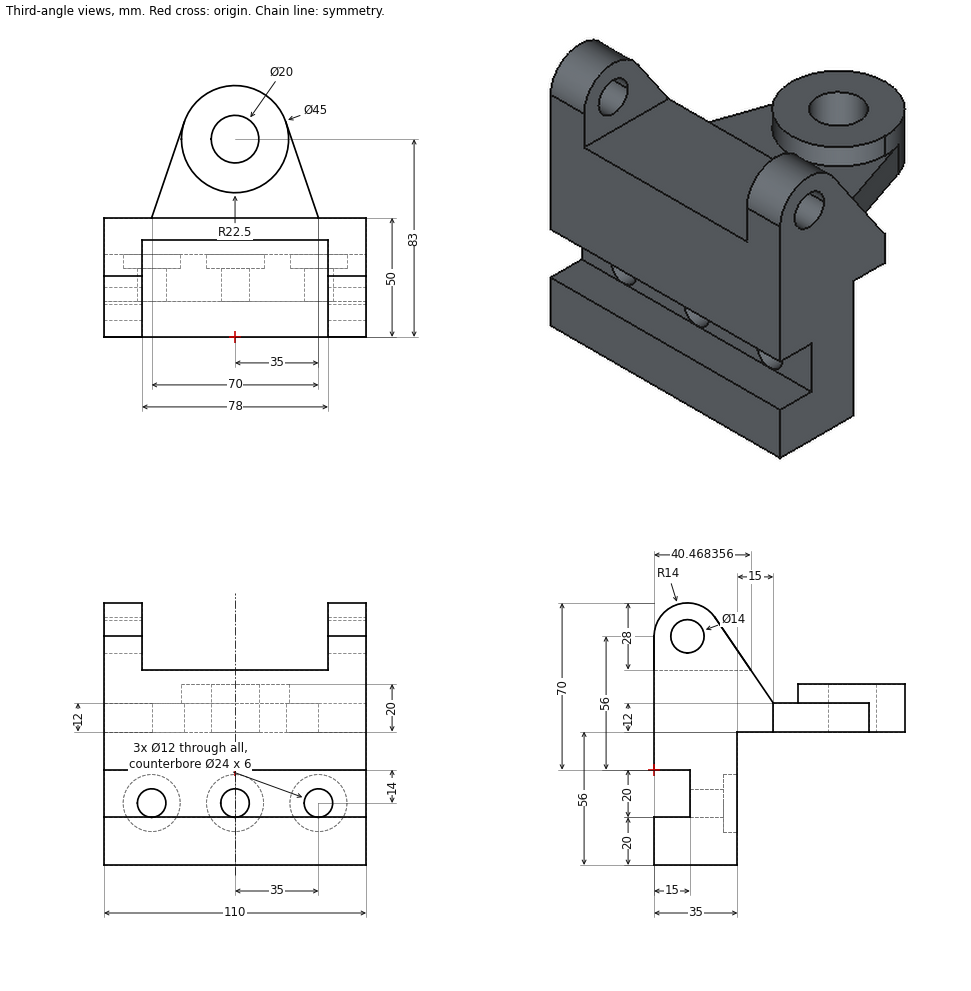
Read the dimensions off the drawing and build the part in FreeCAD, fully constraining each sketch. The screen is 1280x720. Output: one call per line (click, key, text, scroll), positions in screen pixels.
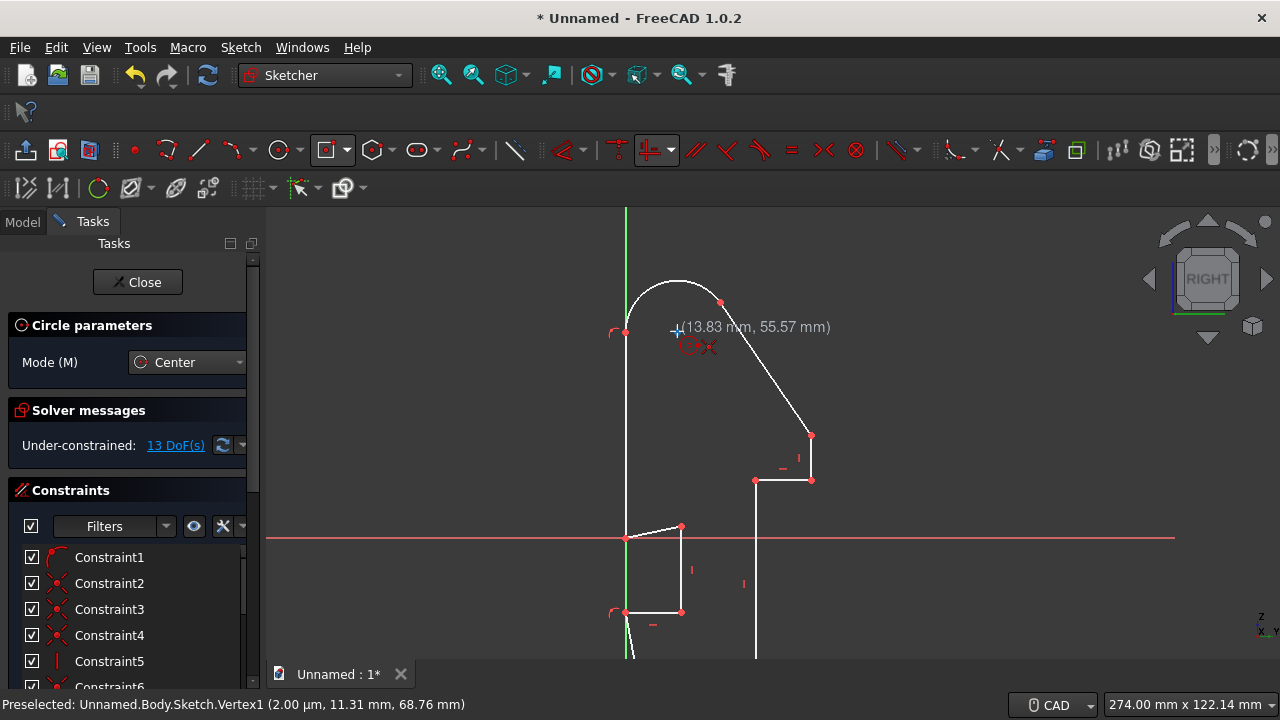
click(677, 331)
click(696, 312)
key(Escape)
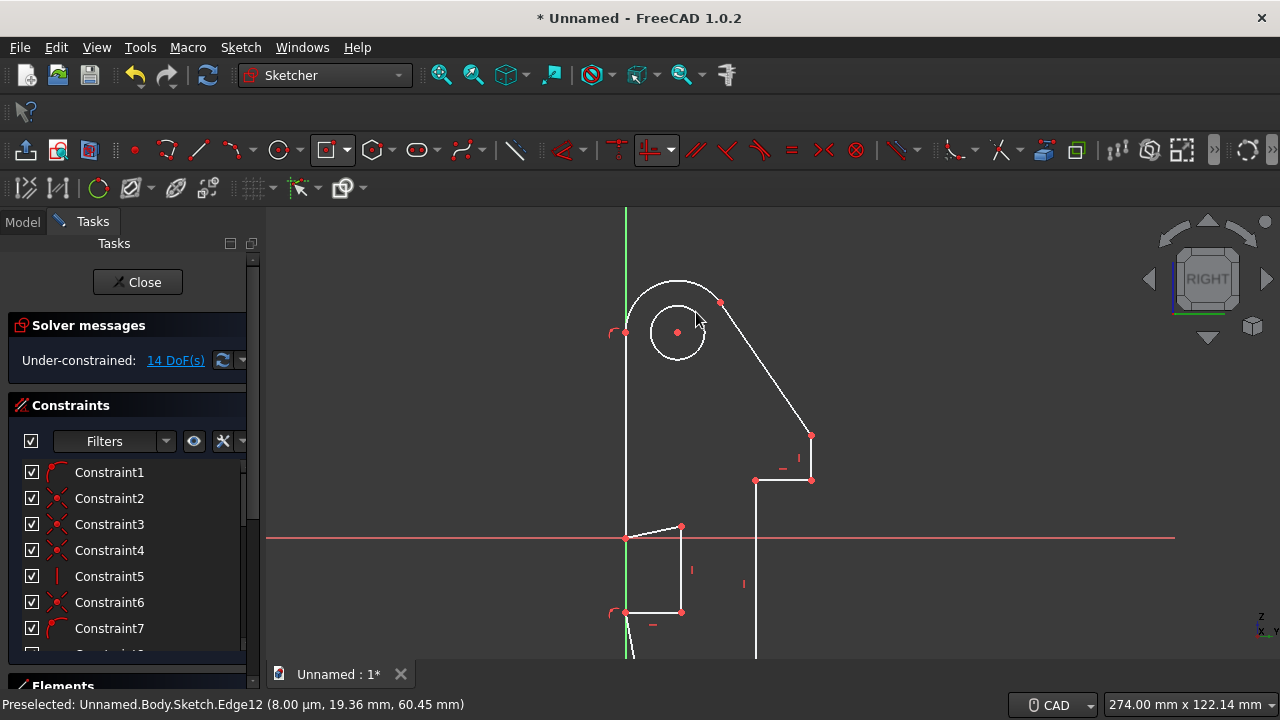
click(626, 394)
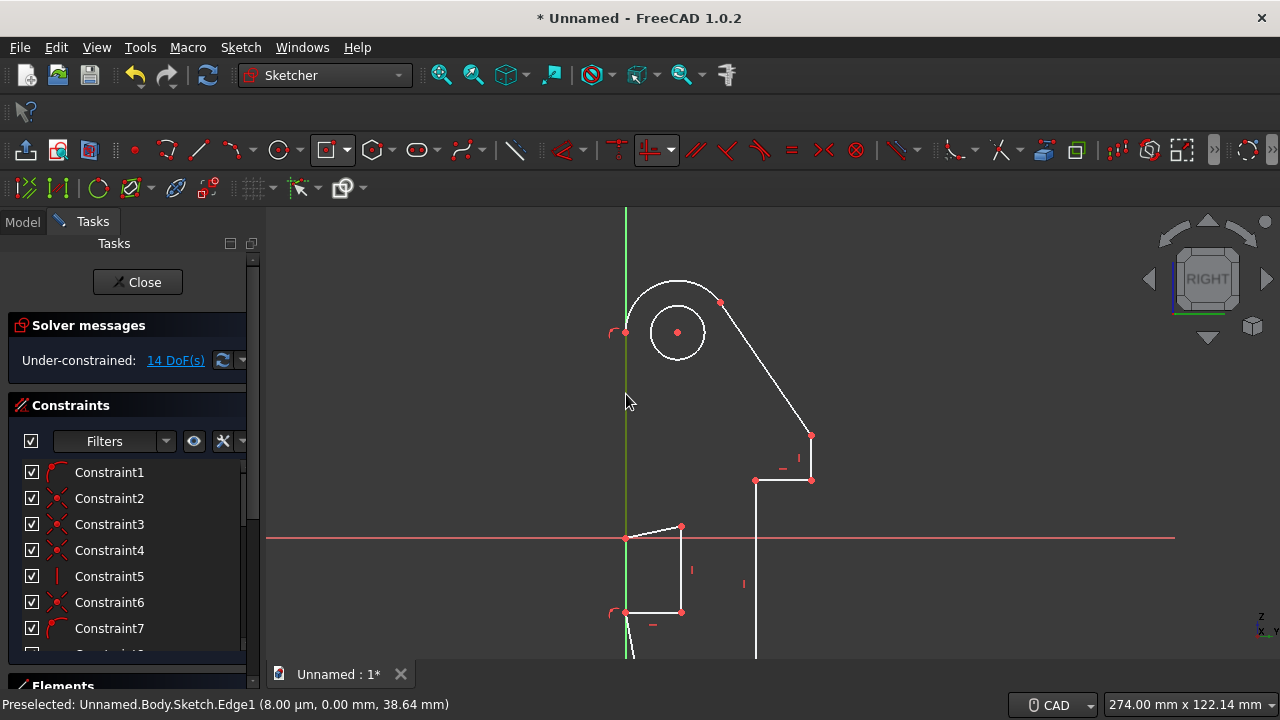
click(688, 282)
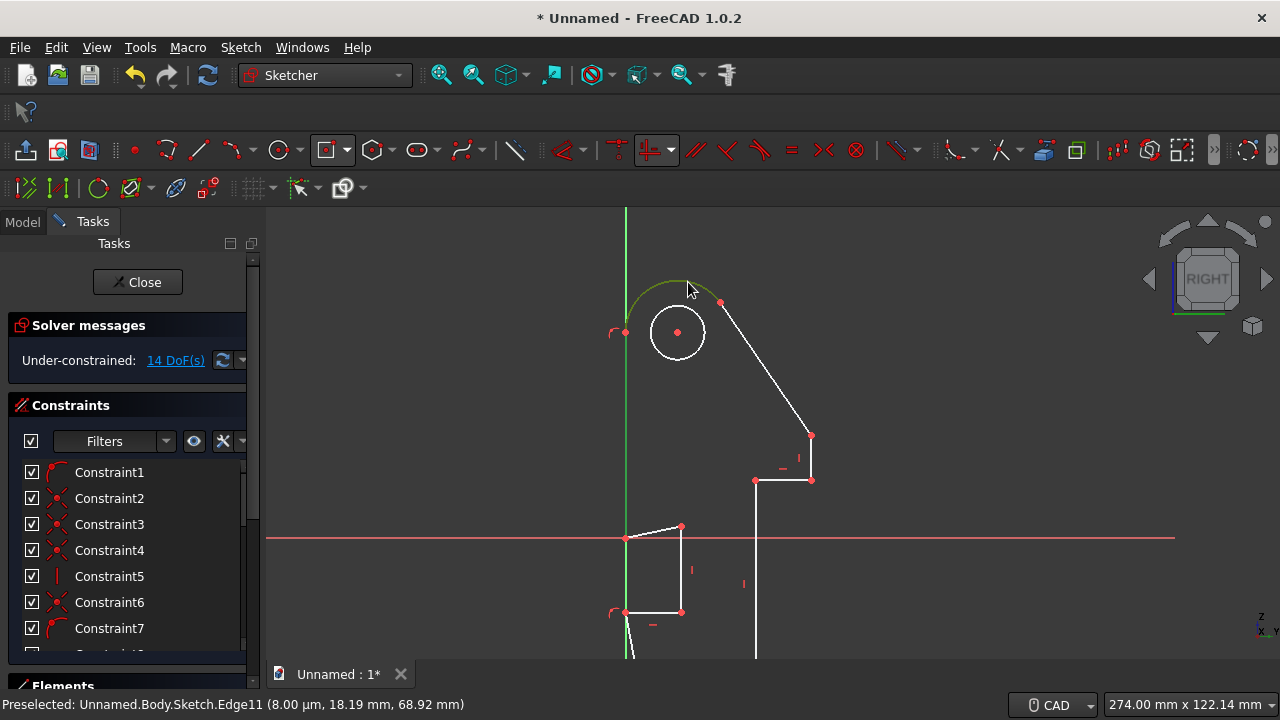
click(760, 150)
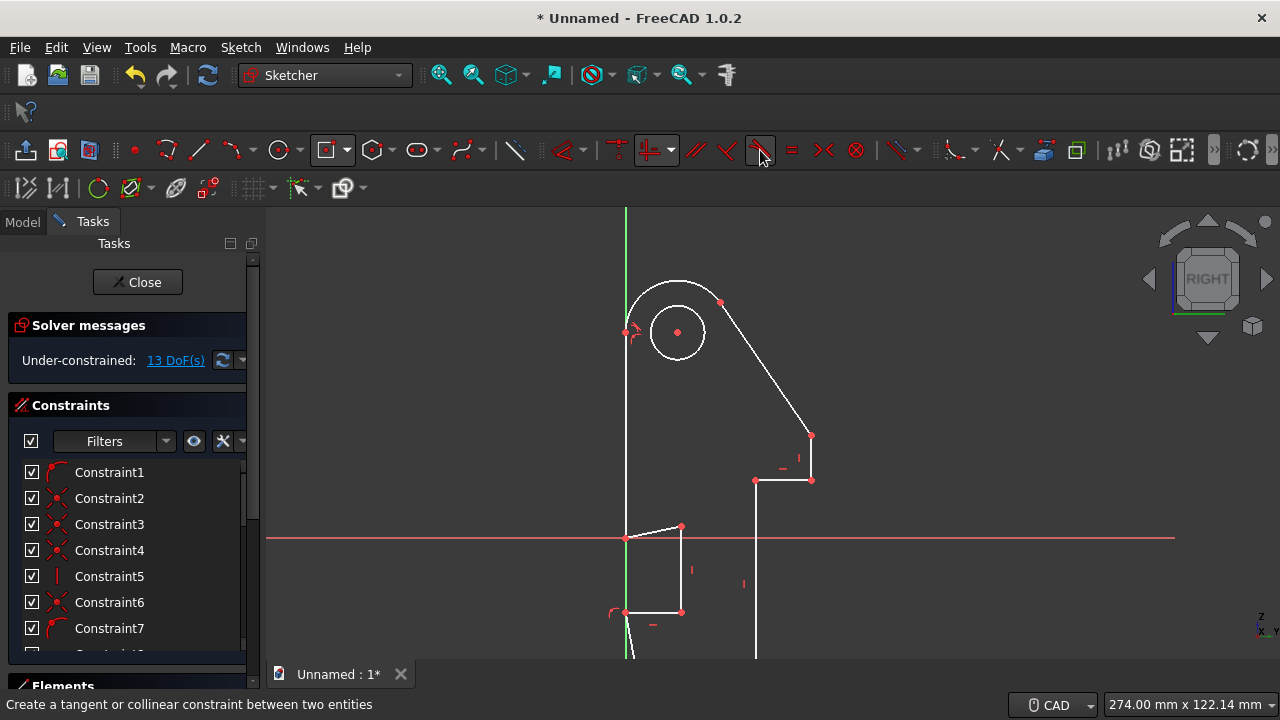
click(784, 395)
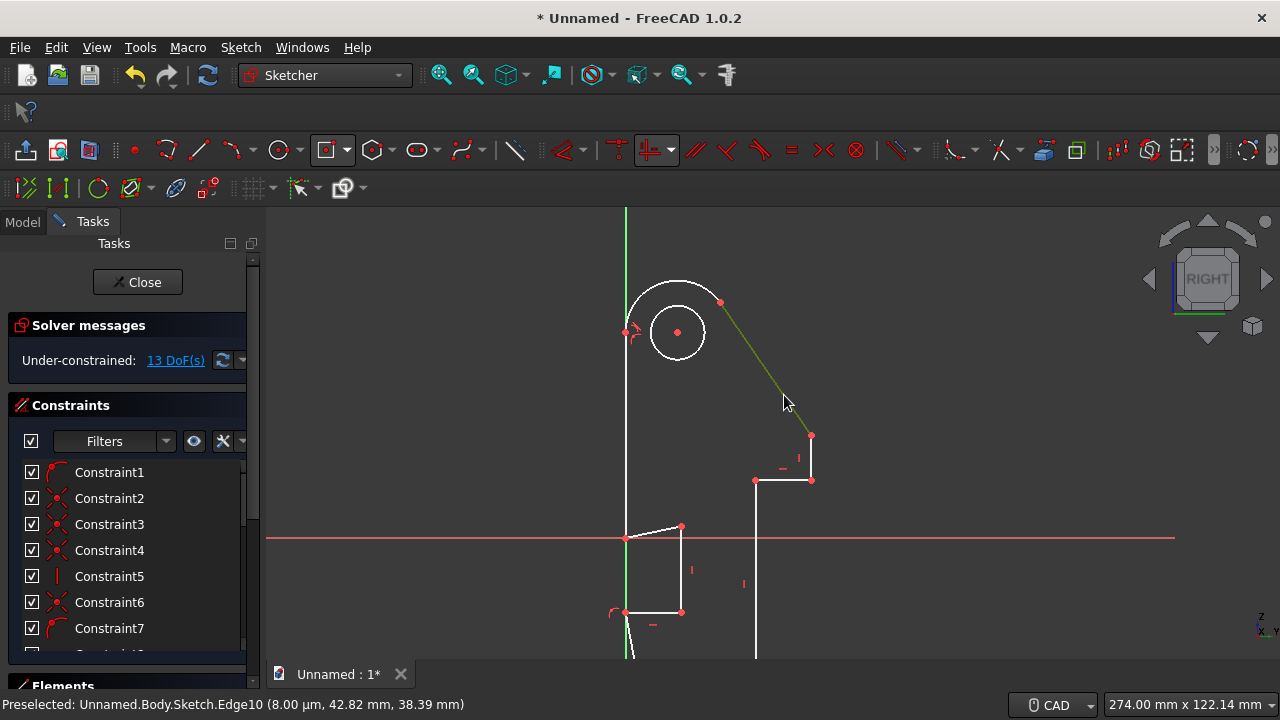
click(688, 282)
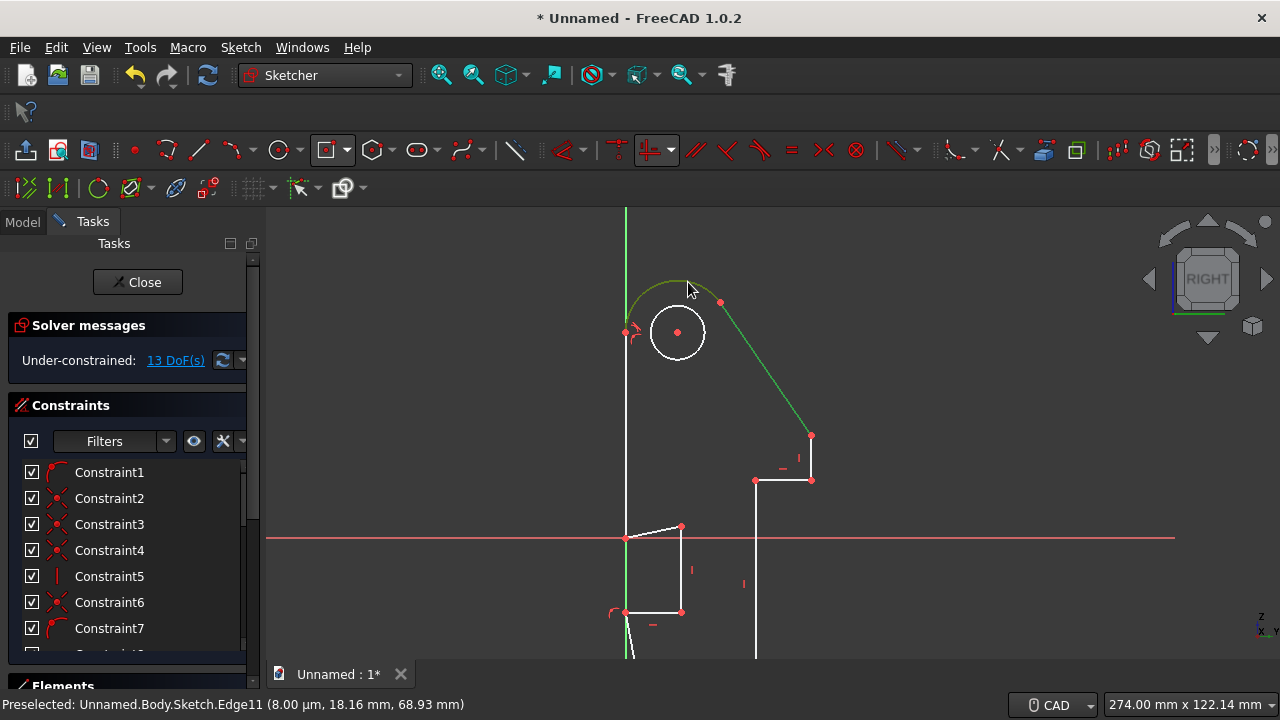
click(760, 150)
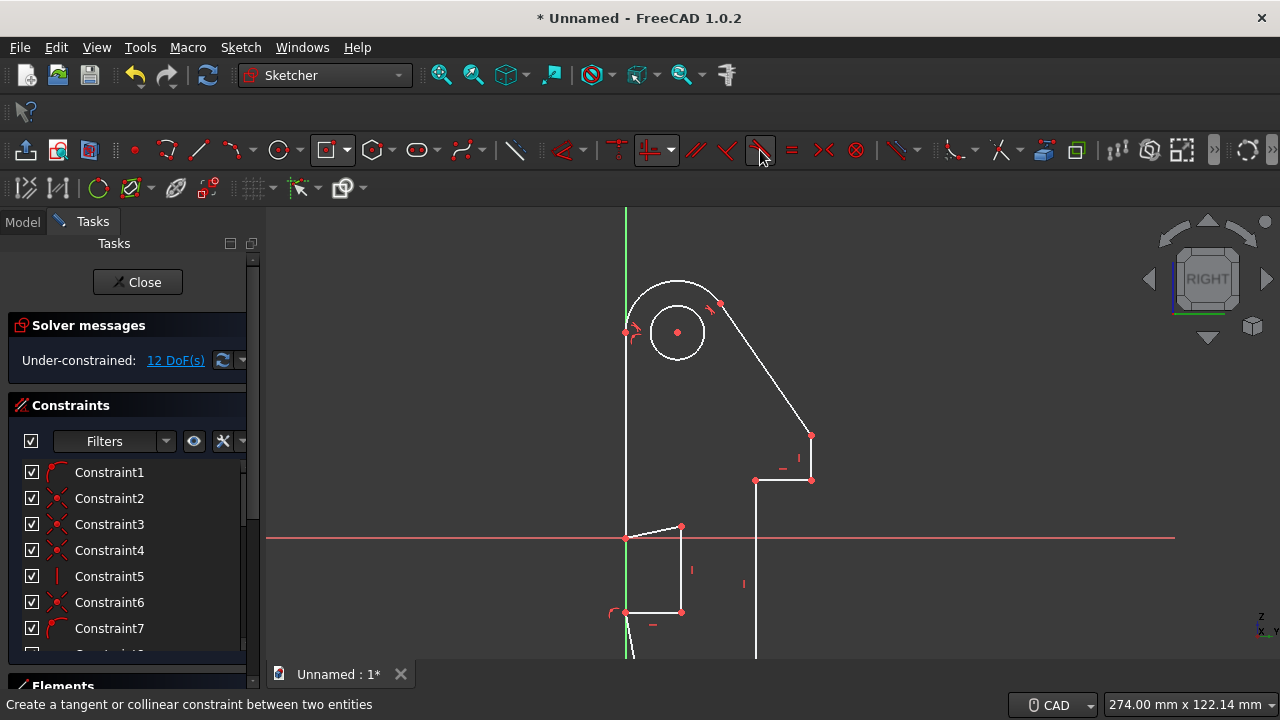
click(642, 534)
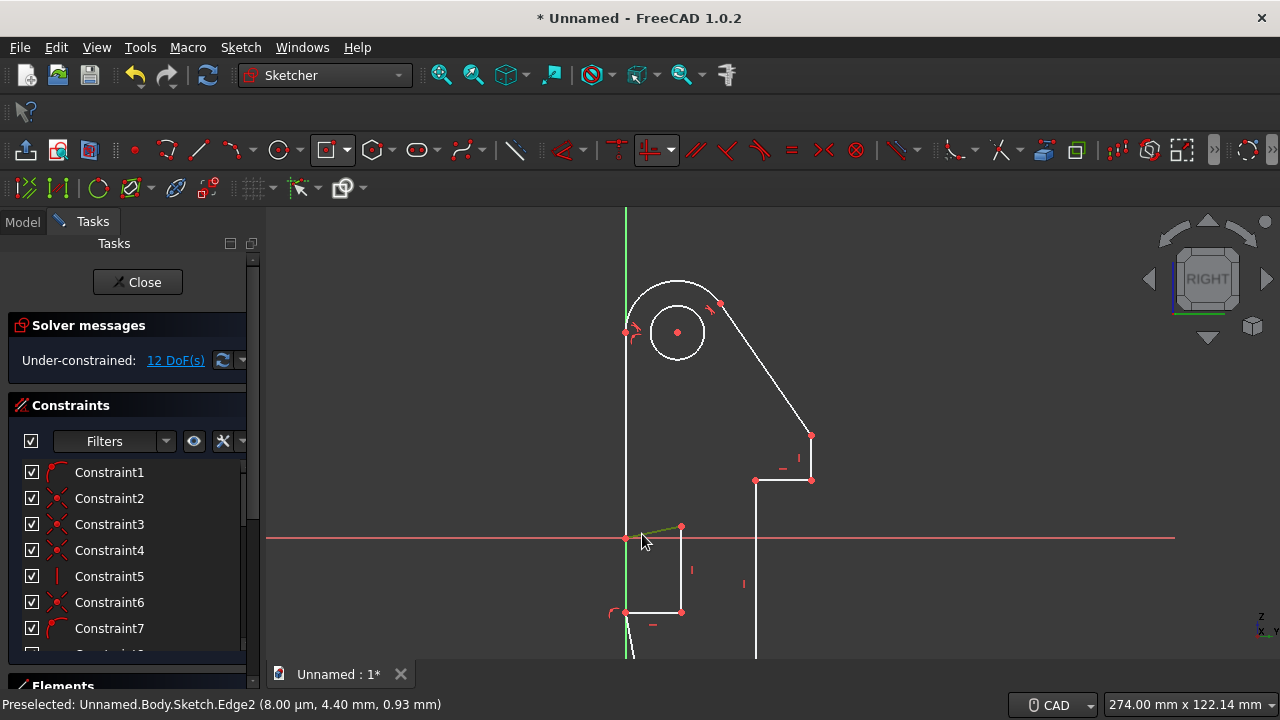
key(h)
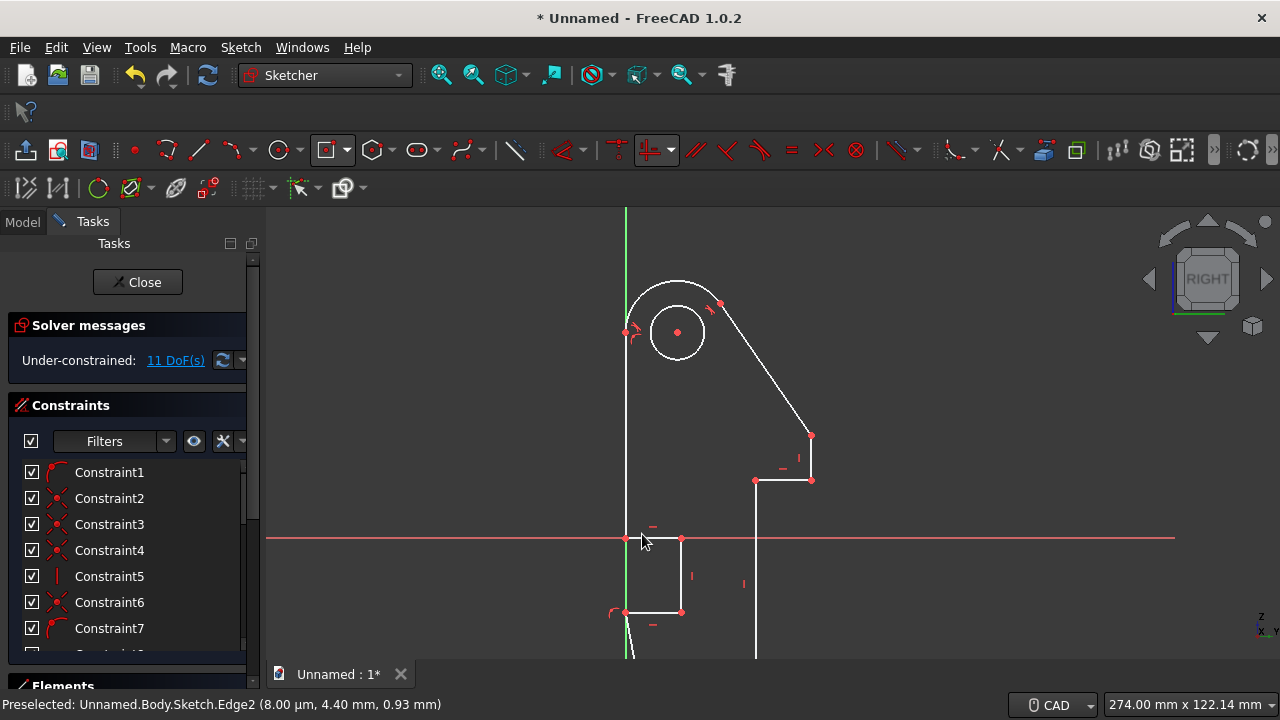
click(628, 628)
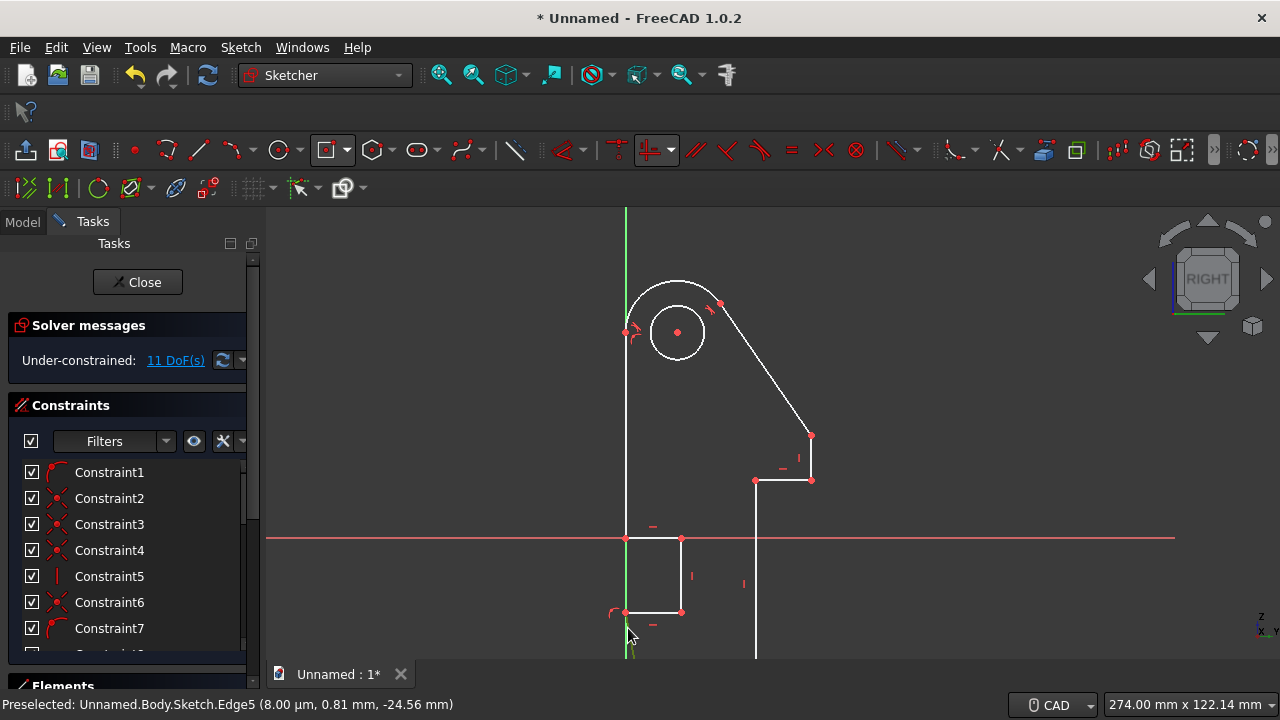
click(674, 150)